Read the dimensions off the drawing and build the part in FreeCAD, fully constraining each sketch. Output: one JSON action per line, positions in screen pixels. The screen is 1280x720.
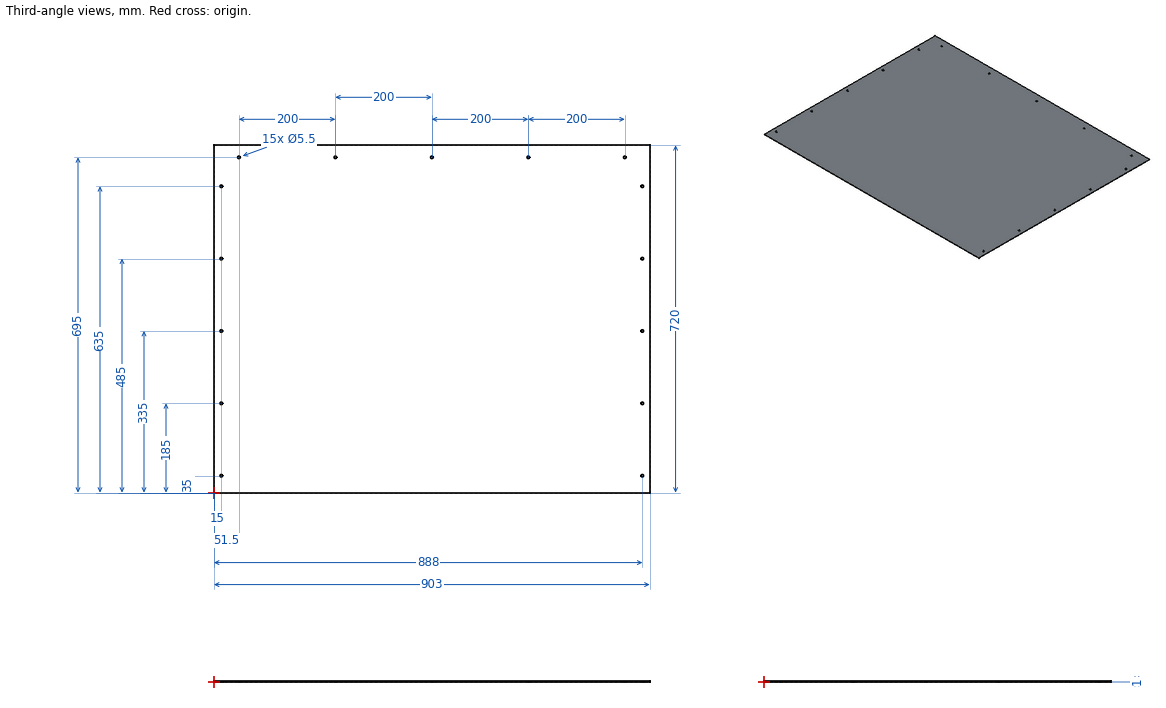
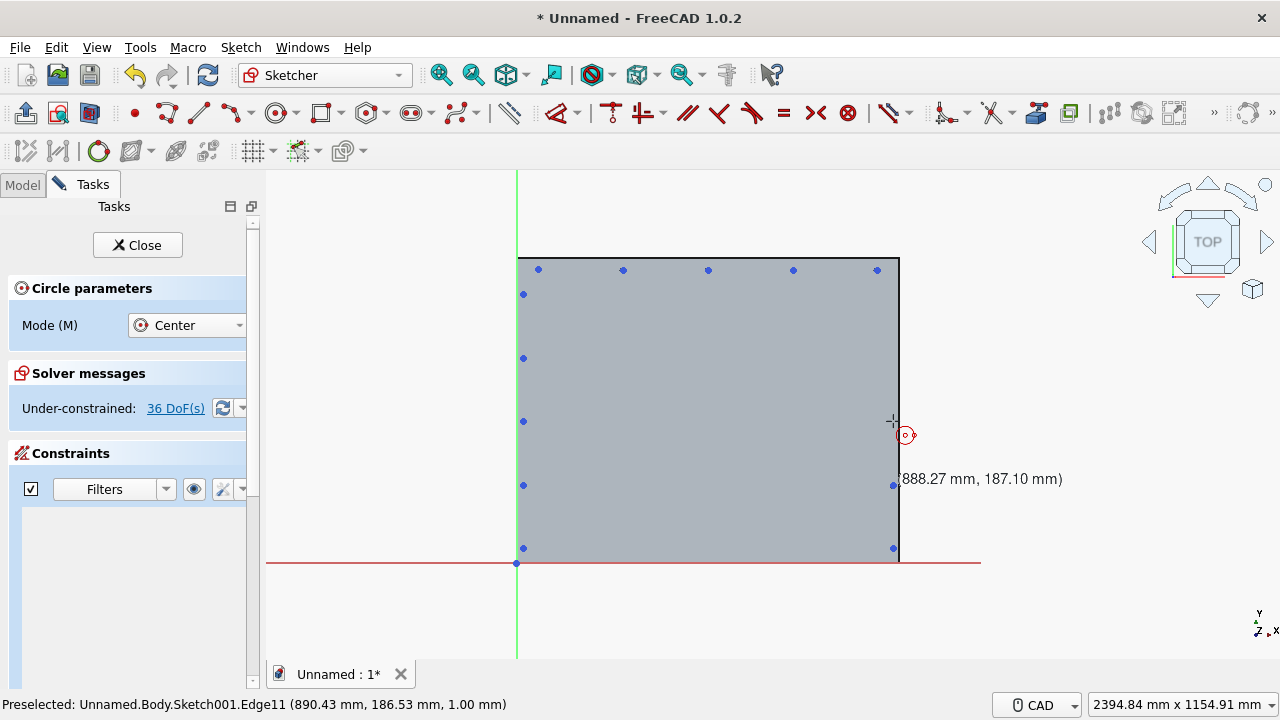
{"action": "left_click", "coordinate": [893, 421]}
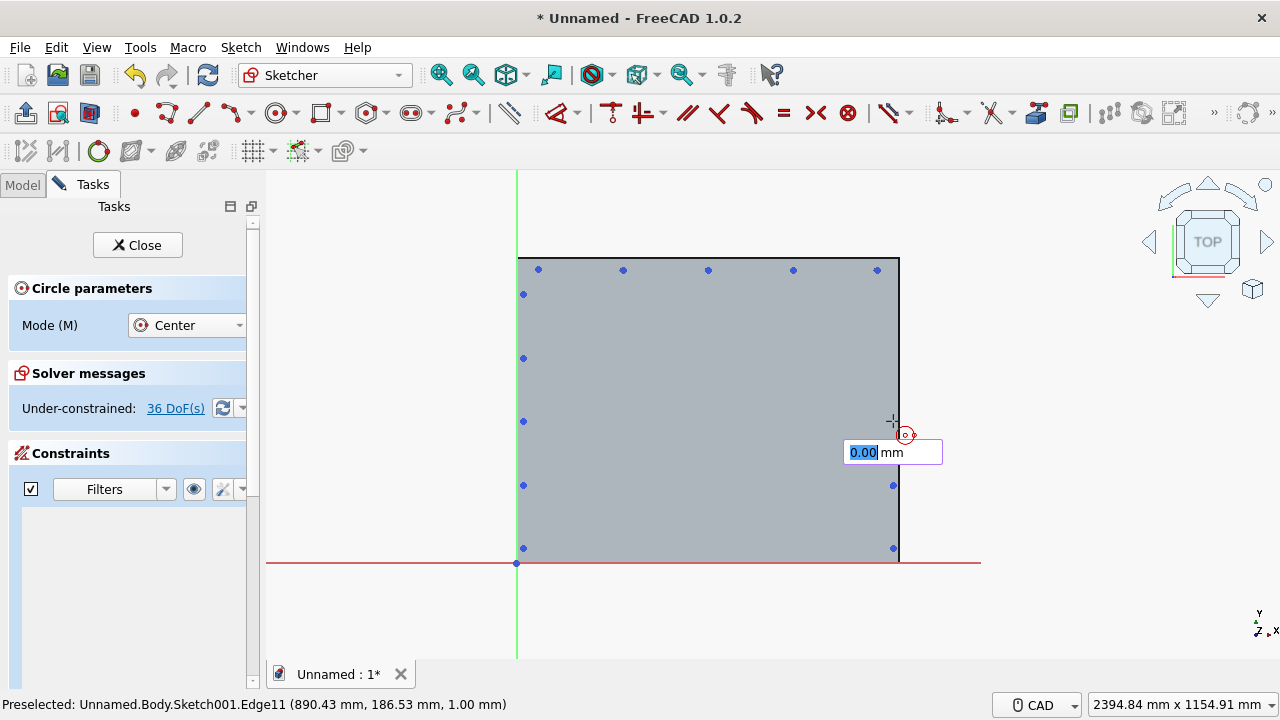
{"action": "scroll", "coordinate": [894, 420], "scroll_direction": "up", "scroll_amount": 14}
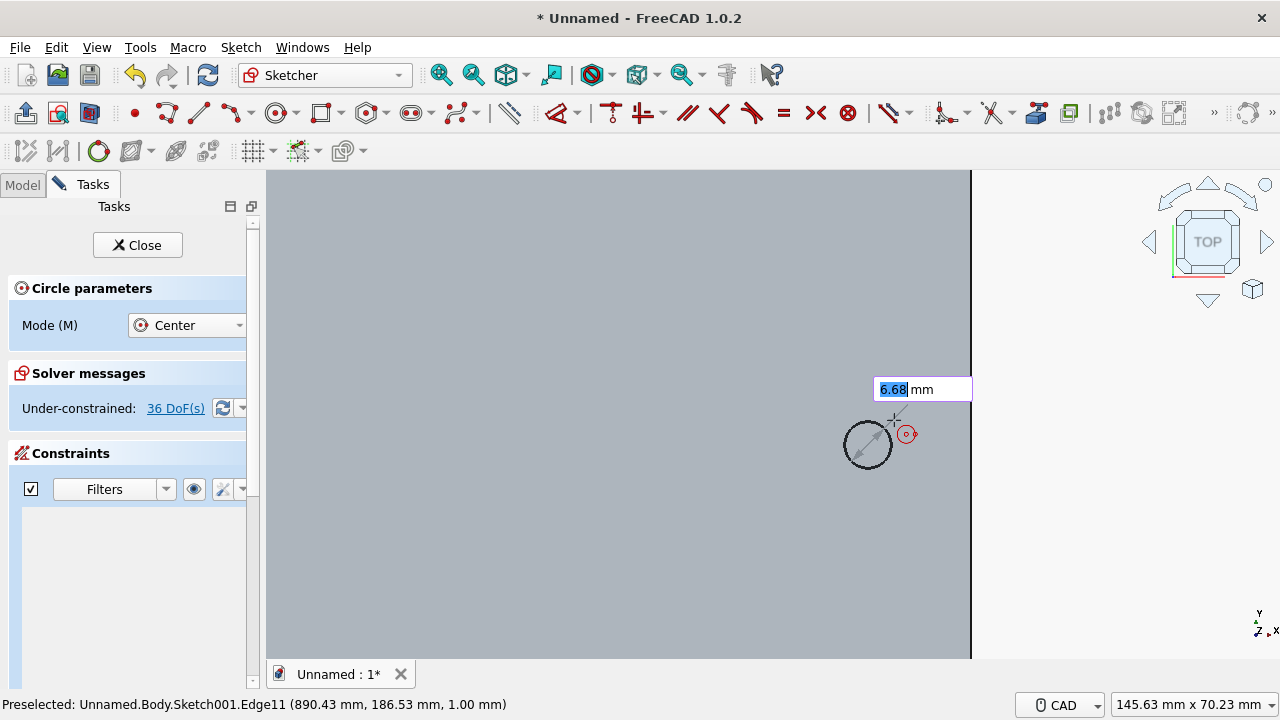
{"action": "left_click", "coordinate": [880, 418]}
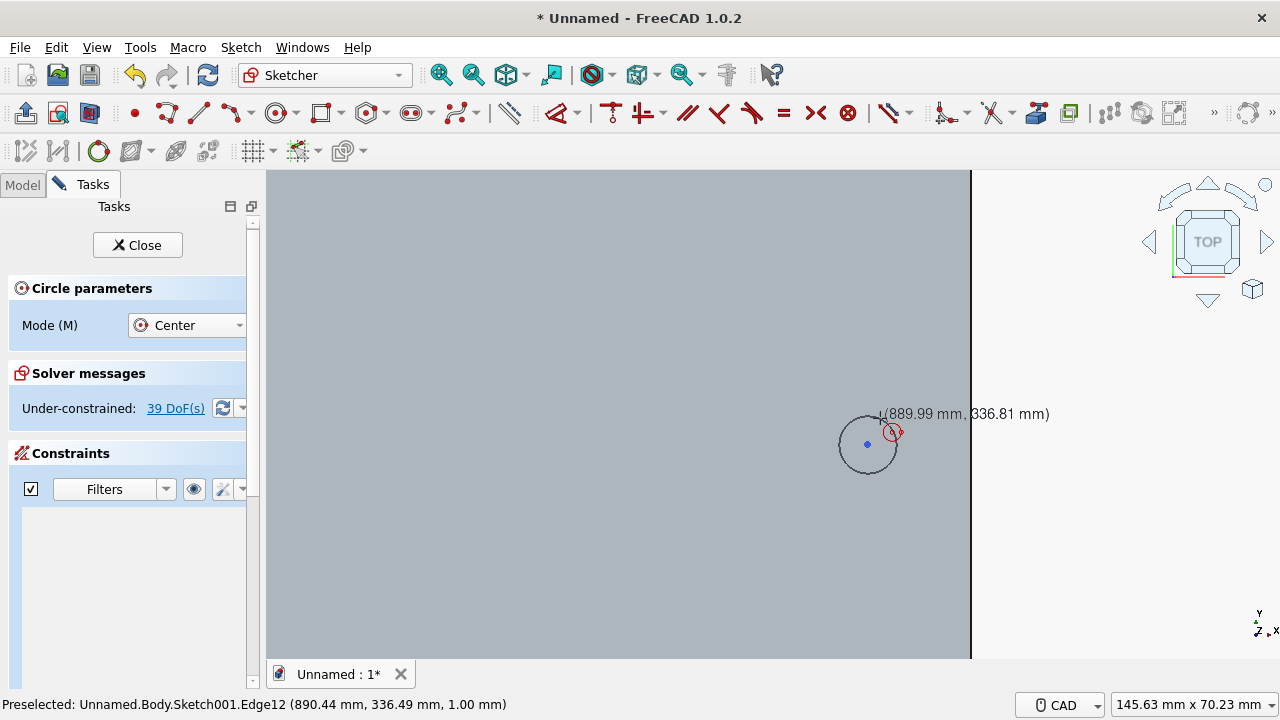
{"action": "scroll", "coordinate": [894, 420], "scroll_direction": "down", "scroll_amount": 14}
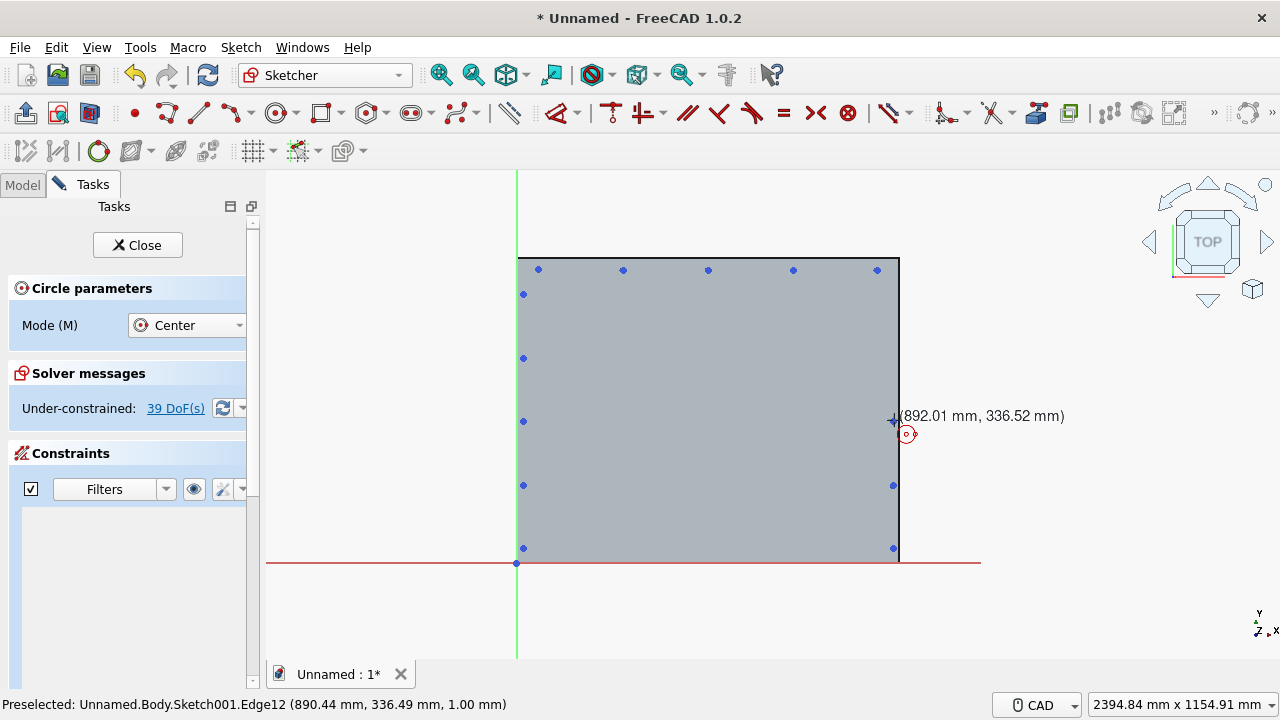
{"action": "scroll", "coordinate": [893, 358], "scroll_direction": "up", "scroll_amount": 15}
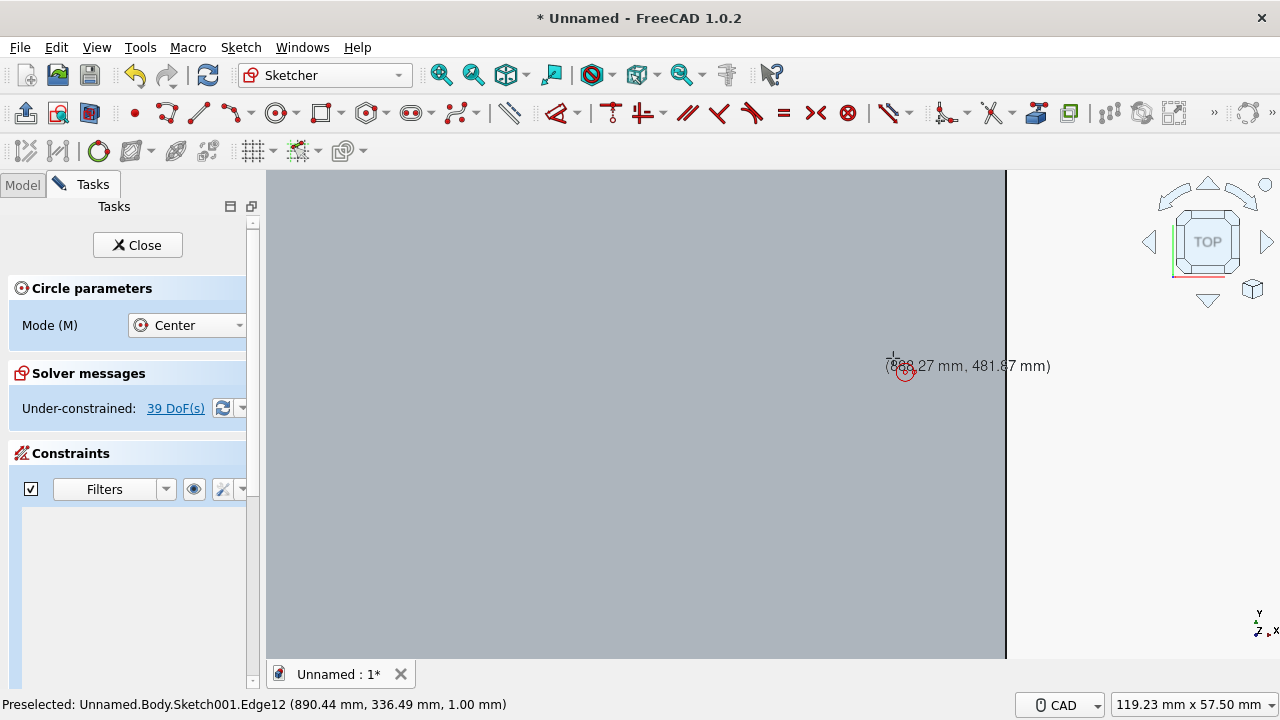
{"action": "scroll", "coordinate": [893, 358], "scroll_direction": "down", "scroll_amount": 15}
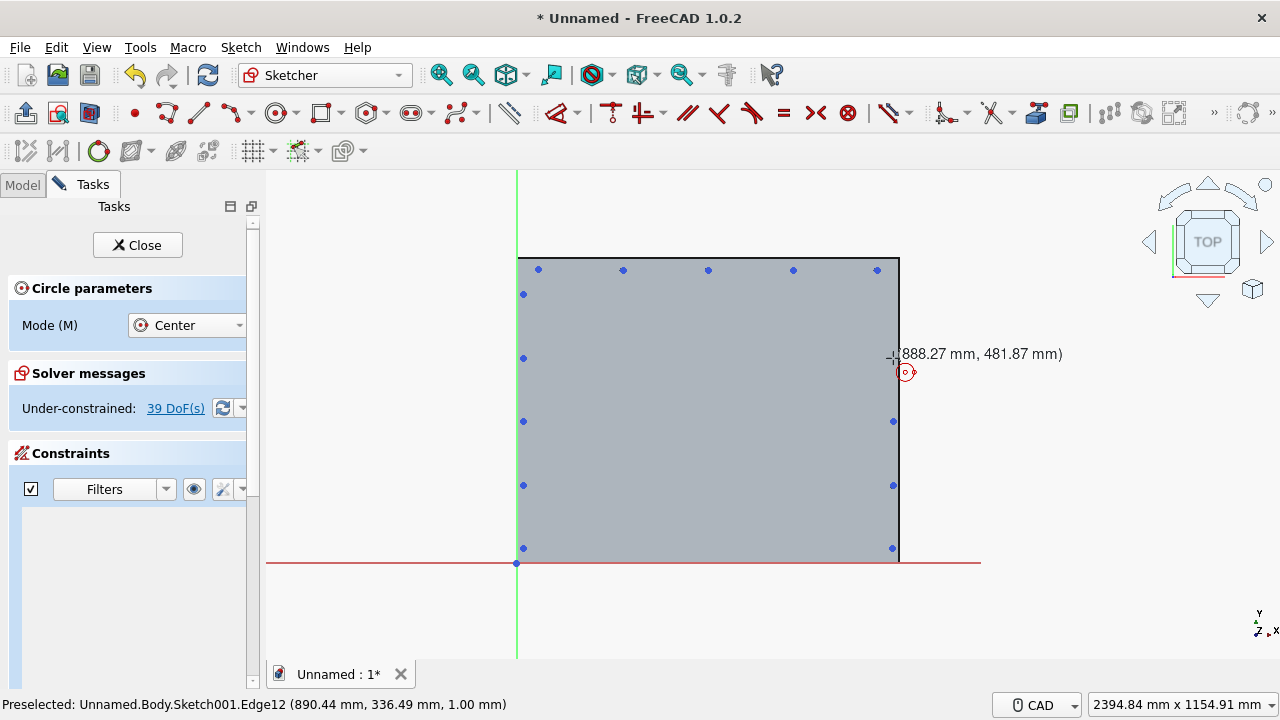
{"action": "left_click", "coordinate": [893, 358]}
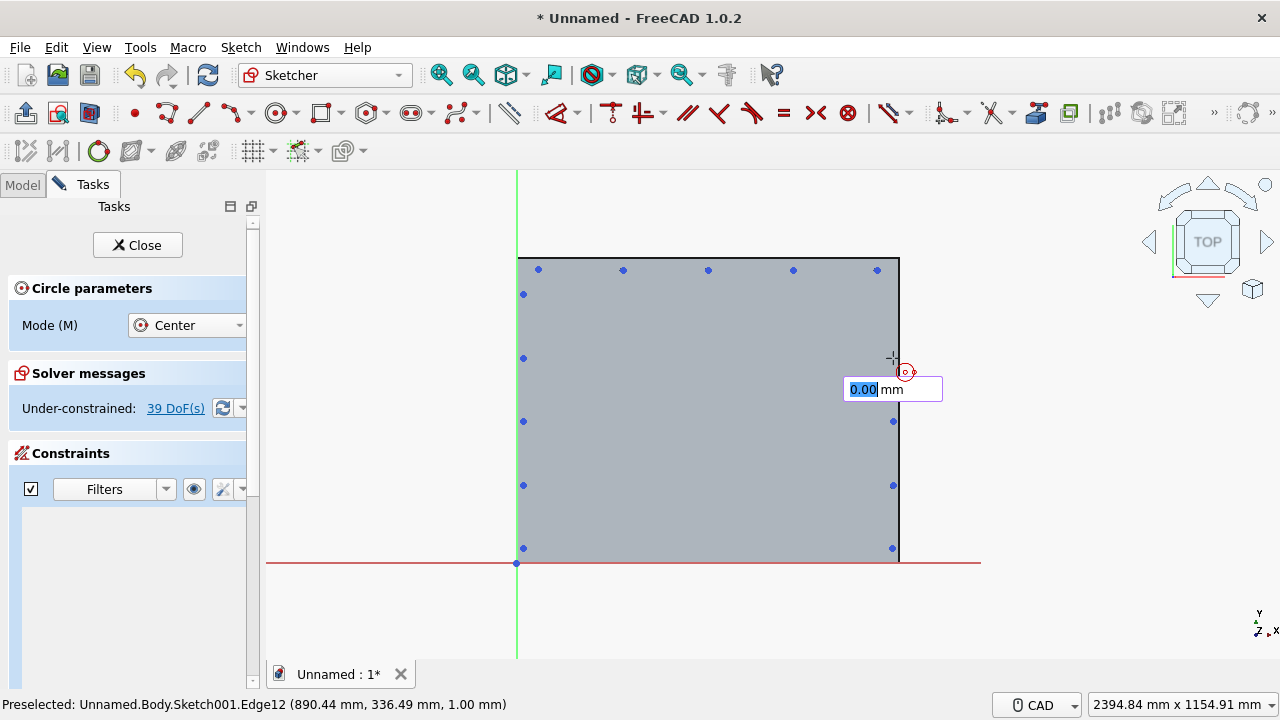
{"action": "scroll", "coordinate": [894, 357], "scroll_direction": "up", "scroll_amount": 14}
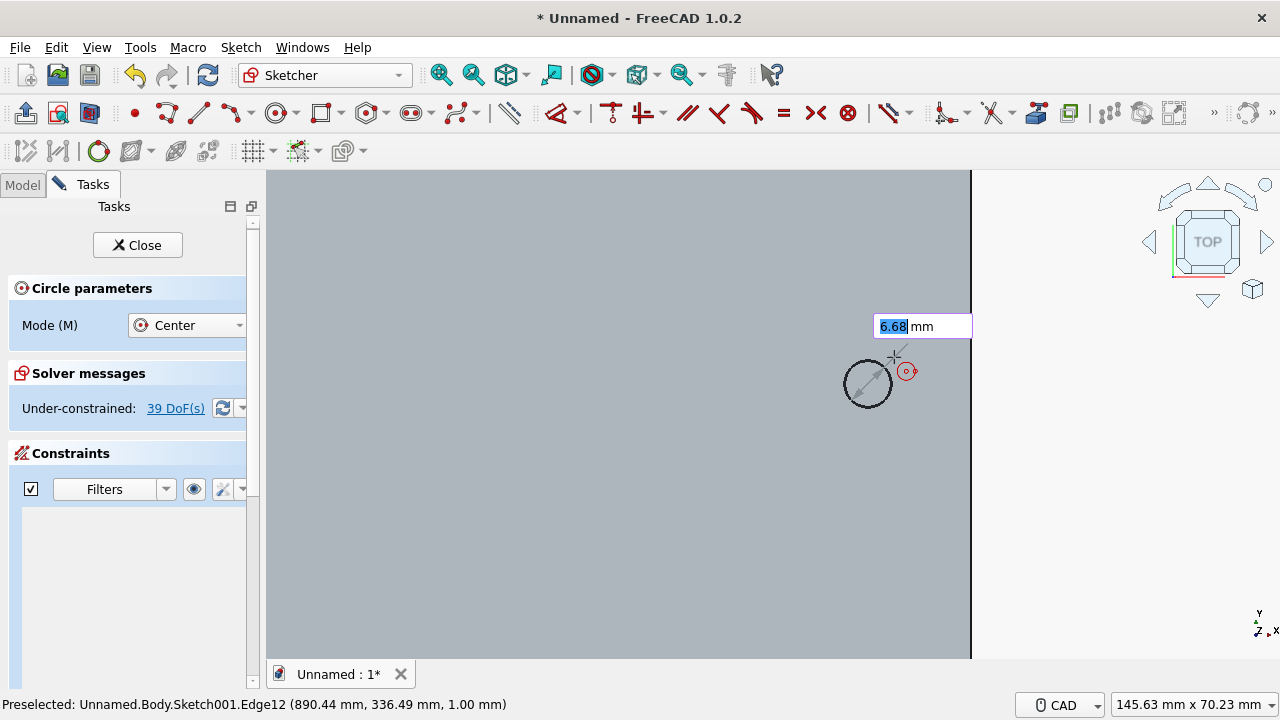
{"action": "left_click", "coordinate": [880, 349]}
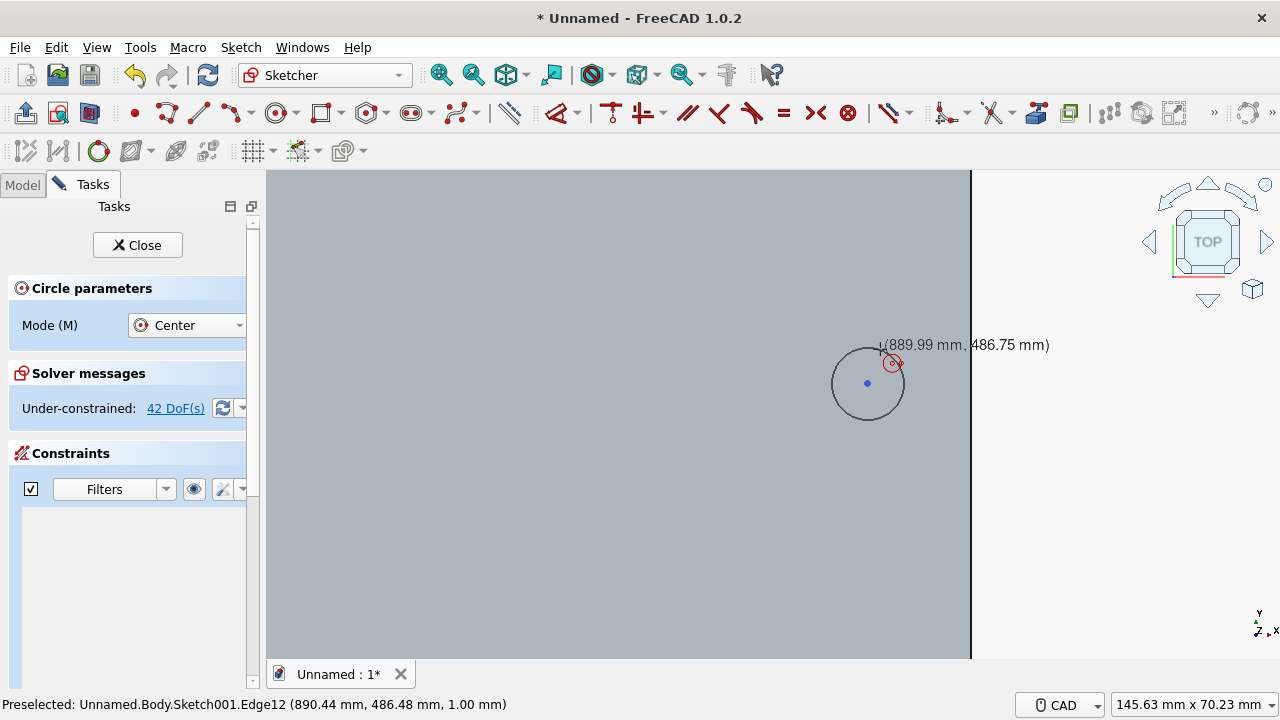
{"action": "scroll", "coordinate": [894, 357], "scroll_direction": "down", "scroll_amount": 14}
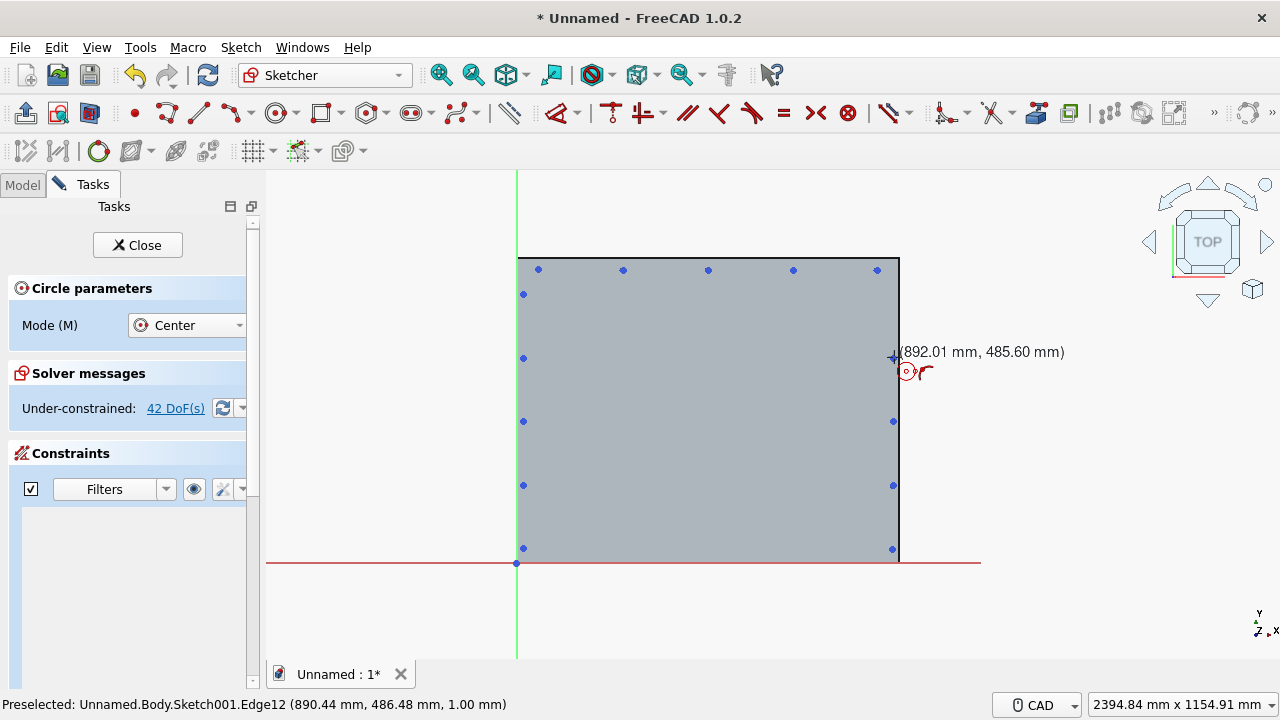
{"action": "scroll", "coordinate": [893, 294], "scroll_direction": "up", "scroll_amount": 15}